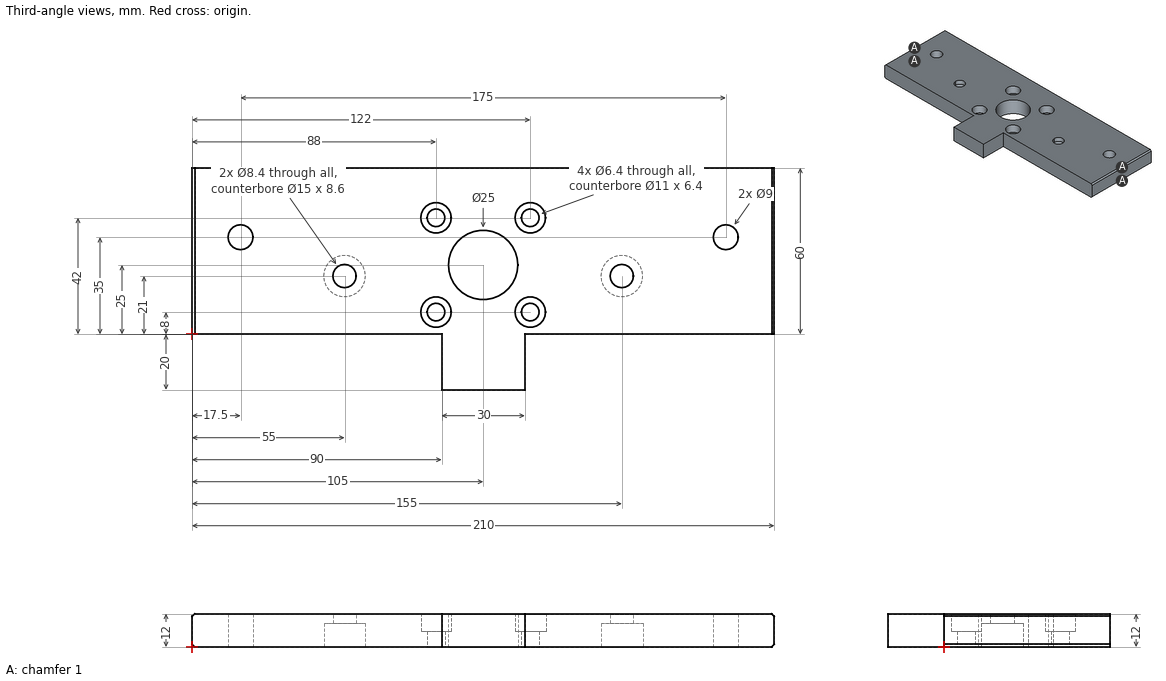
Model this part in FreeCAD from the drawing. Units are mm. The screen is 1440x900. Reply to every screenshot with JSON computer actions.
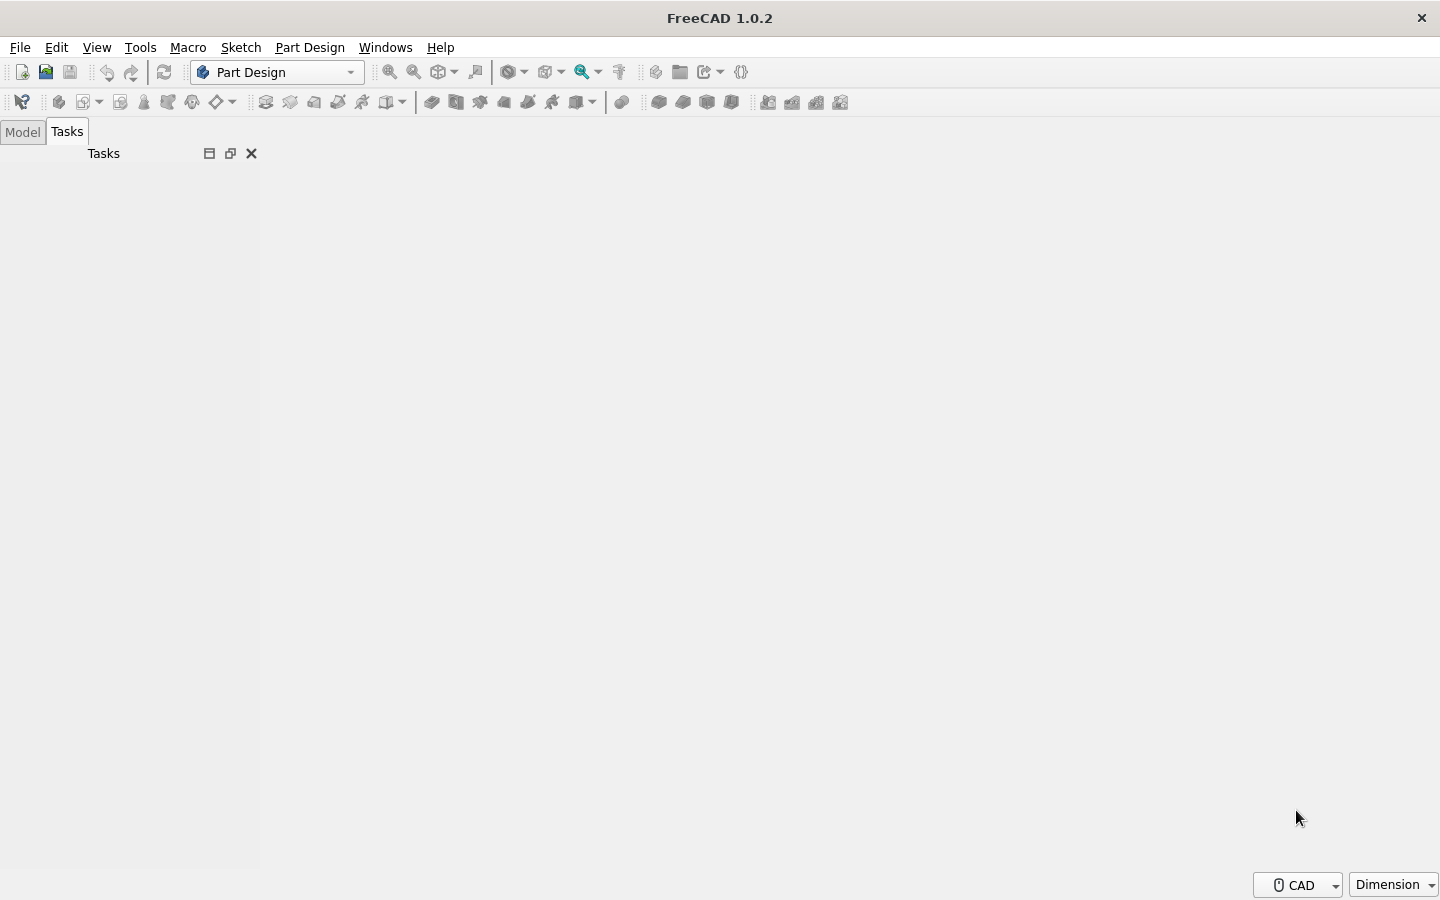
{"action": "key", "text": "ctrl+n"}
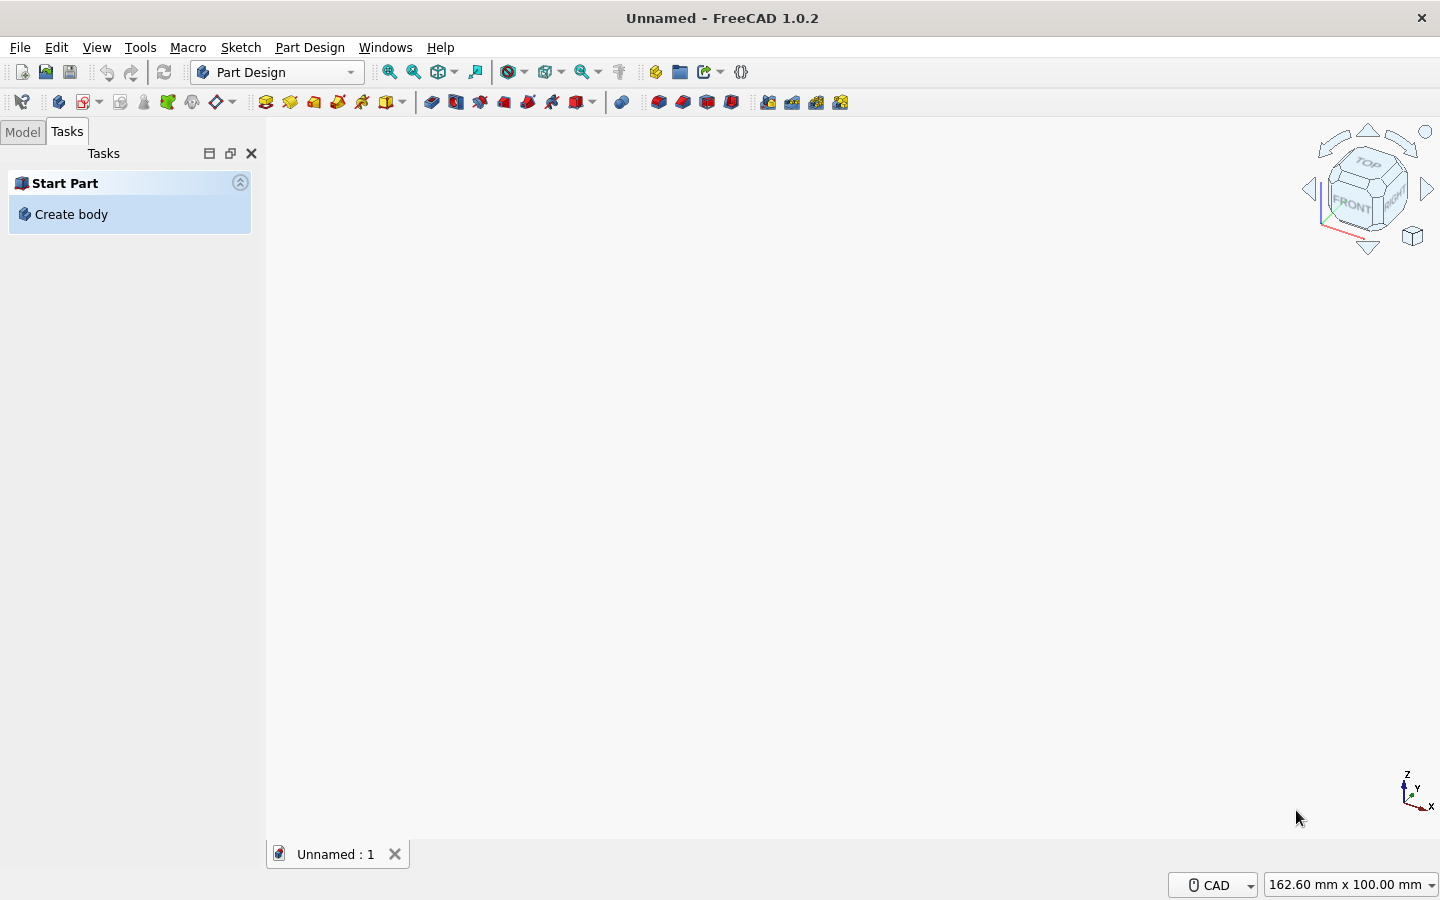
{"action": "left_click", "coordinate": [84, 102]}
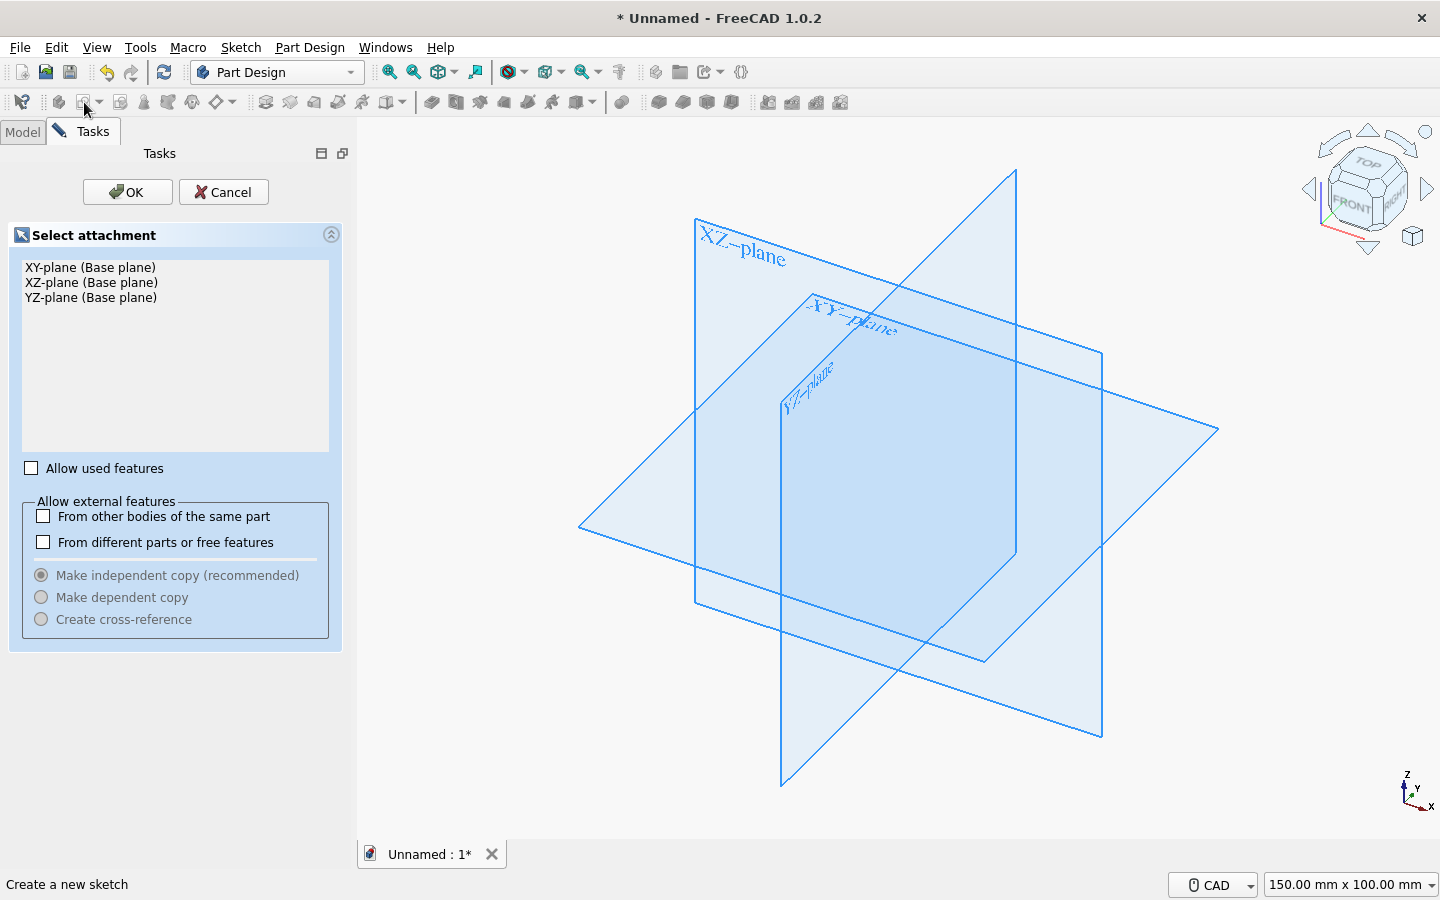
{"action": "left_click", "coordinate": [82, 268]}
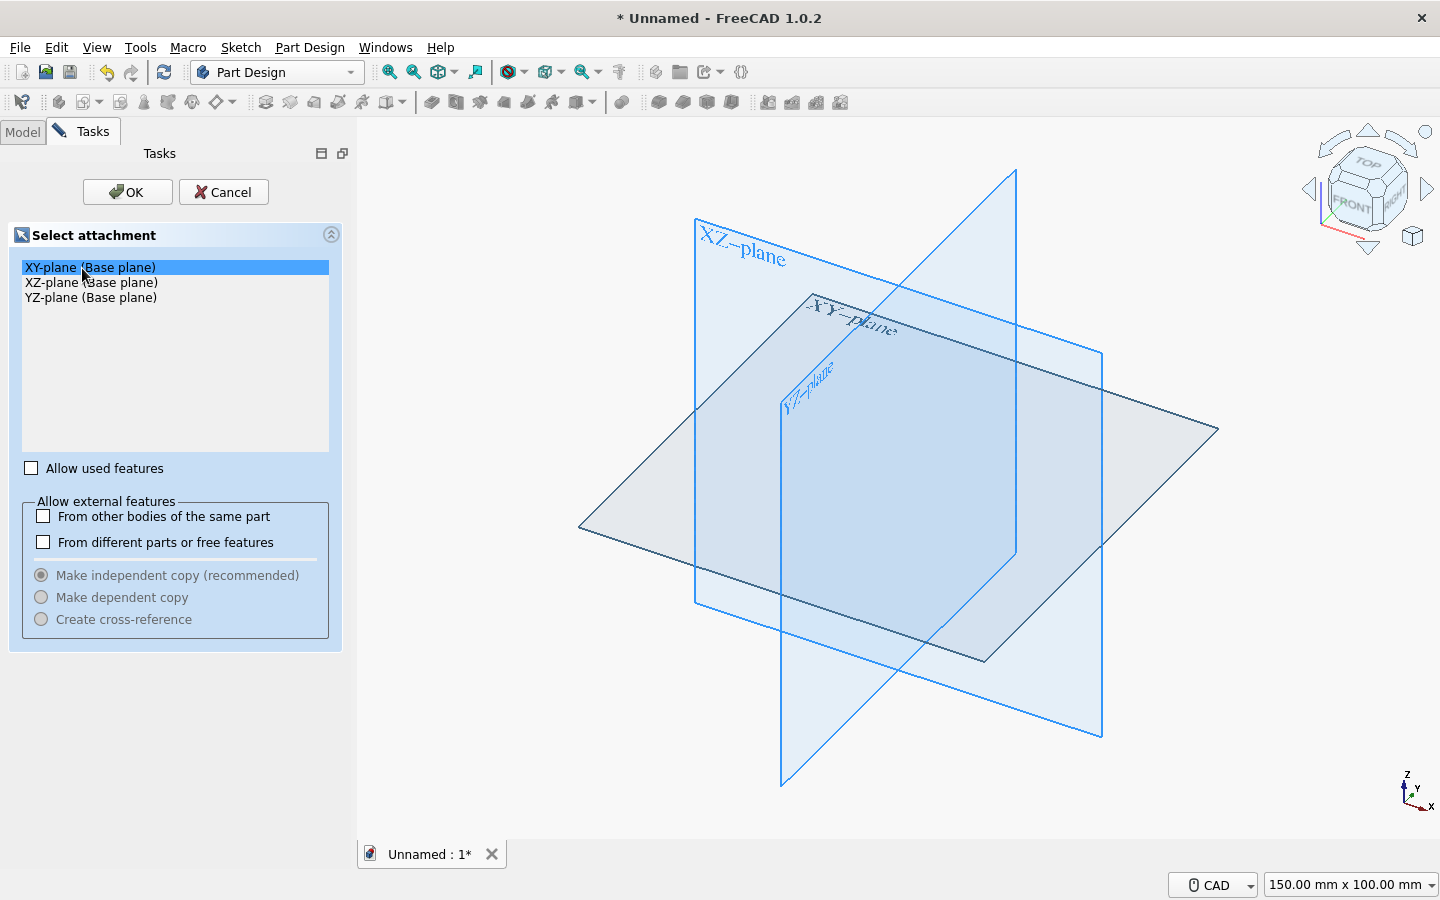
{"action": "left_click", "coordinate": [128, 192]}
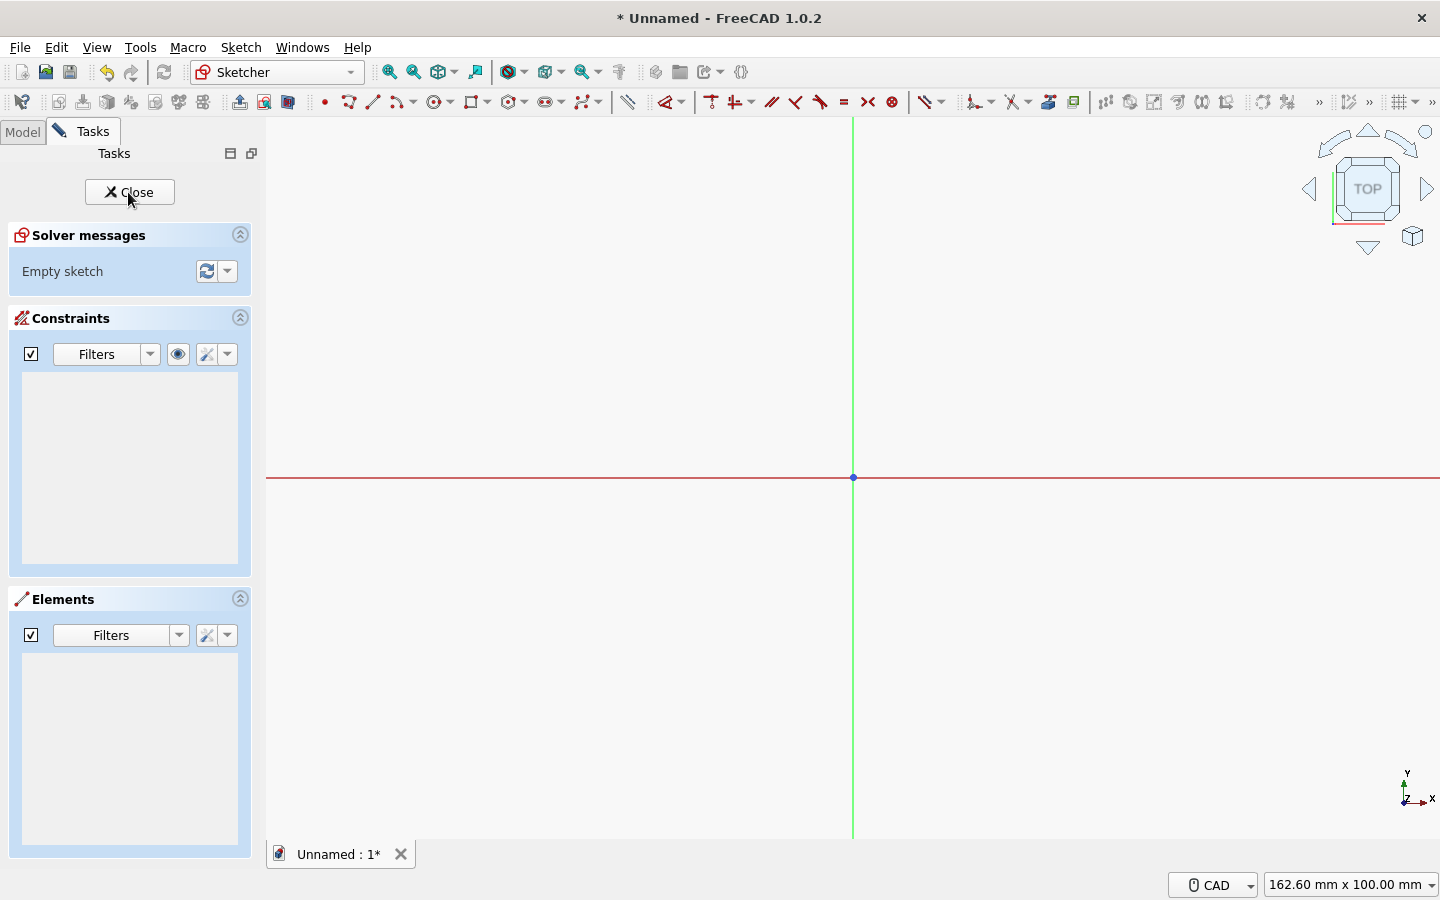
{"action": "scroll", "coordinate": [294, 655], "scroll_direction": "down", "scroll_amount": 4}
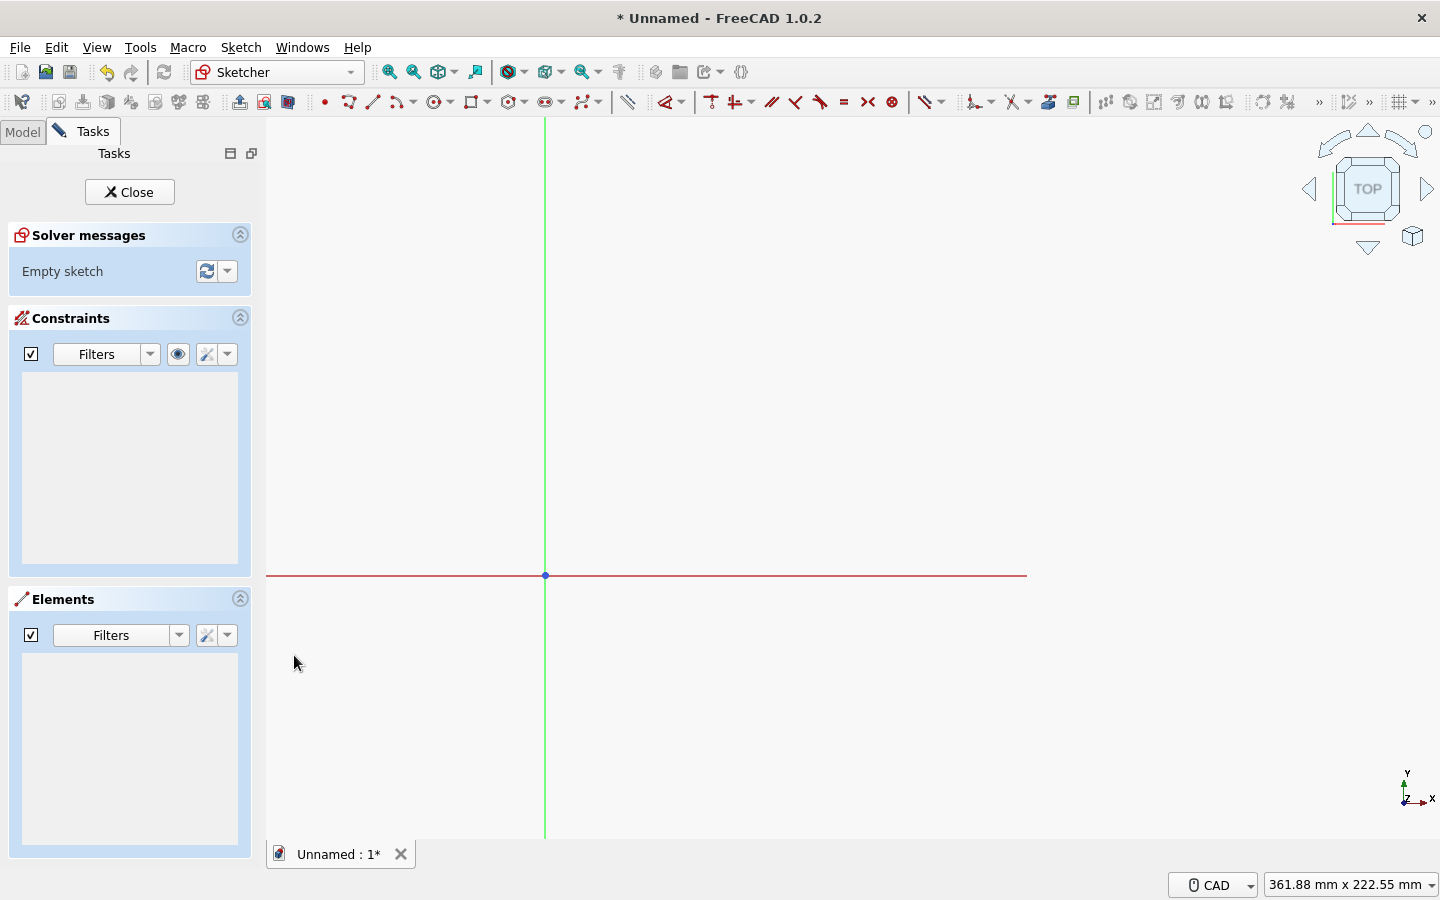
{"action": "left_click", "coordinate": [472, 102]}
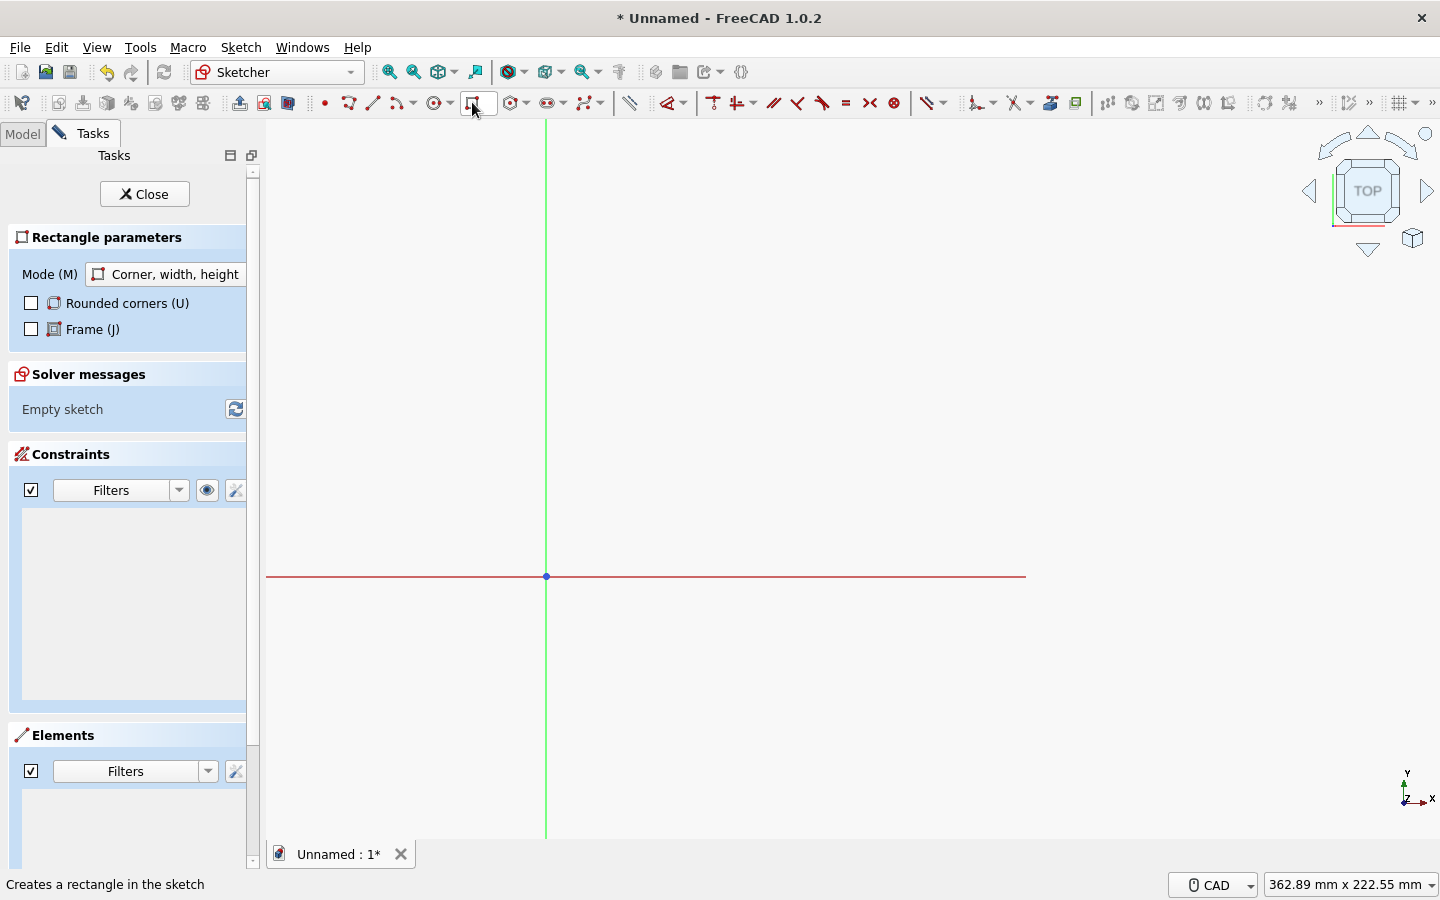
{"action": "left_click", "coordinate": [546, 577]}
{"action": "left_click", "coordinate": [1225, 382]}
{"action": "key", "text": "Escape"}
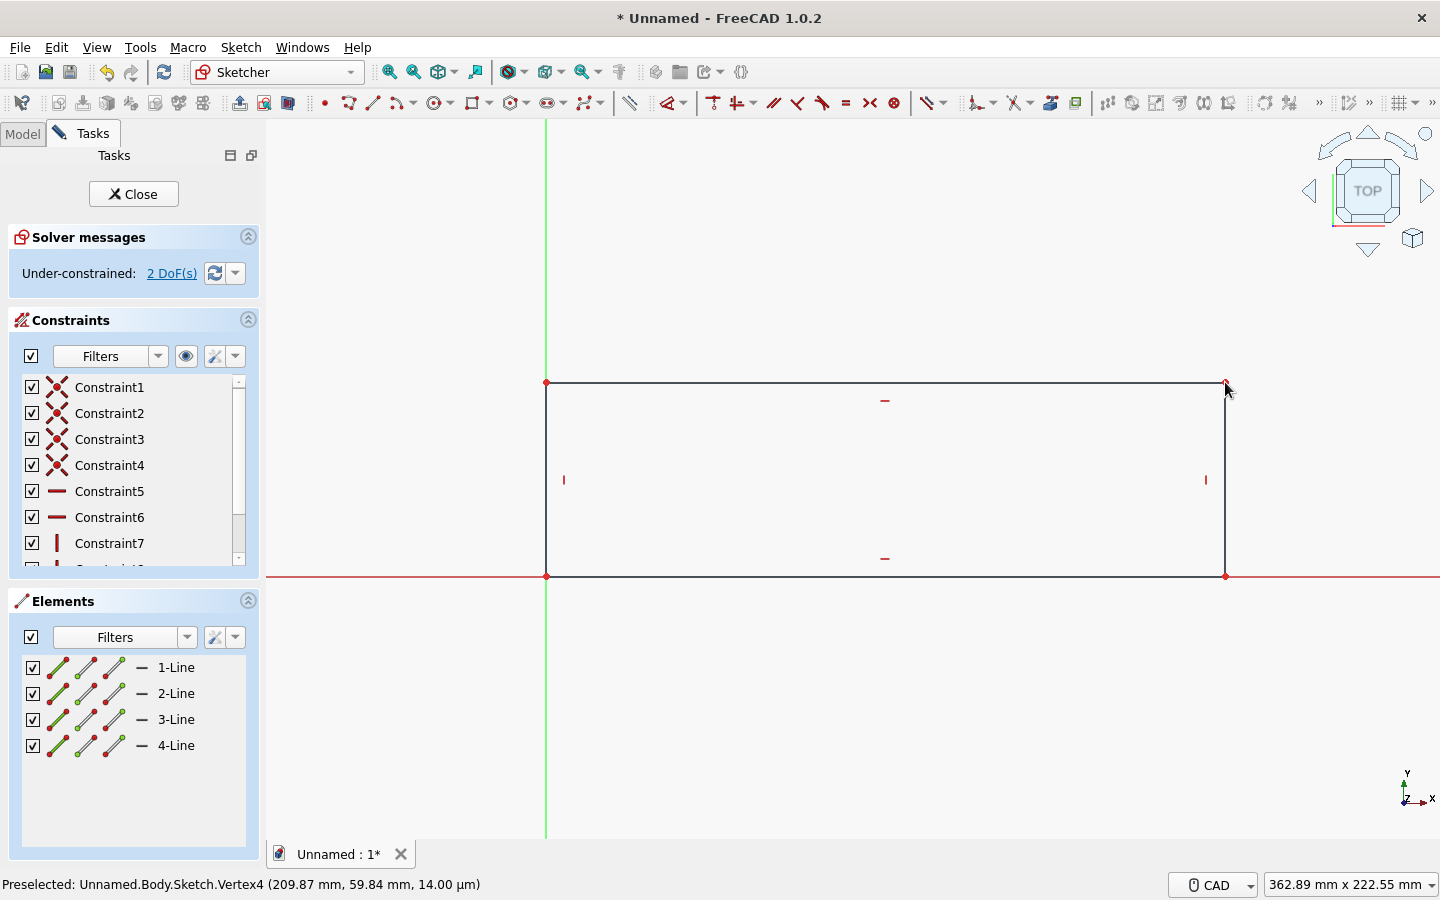
{"action": "left_click", "coordinate": [668, 104]}